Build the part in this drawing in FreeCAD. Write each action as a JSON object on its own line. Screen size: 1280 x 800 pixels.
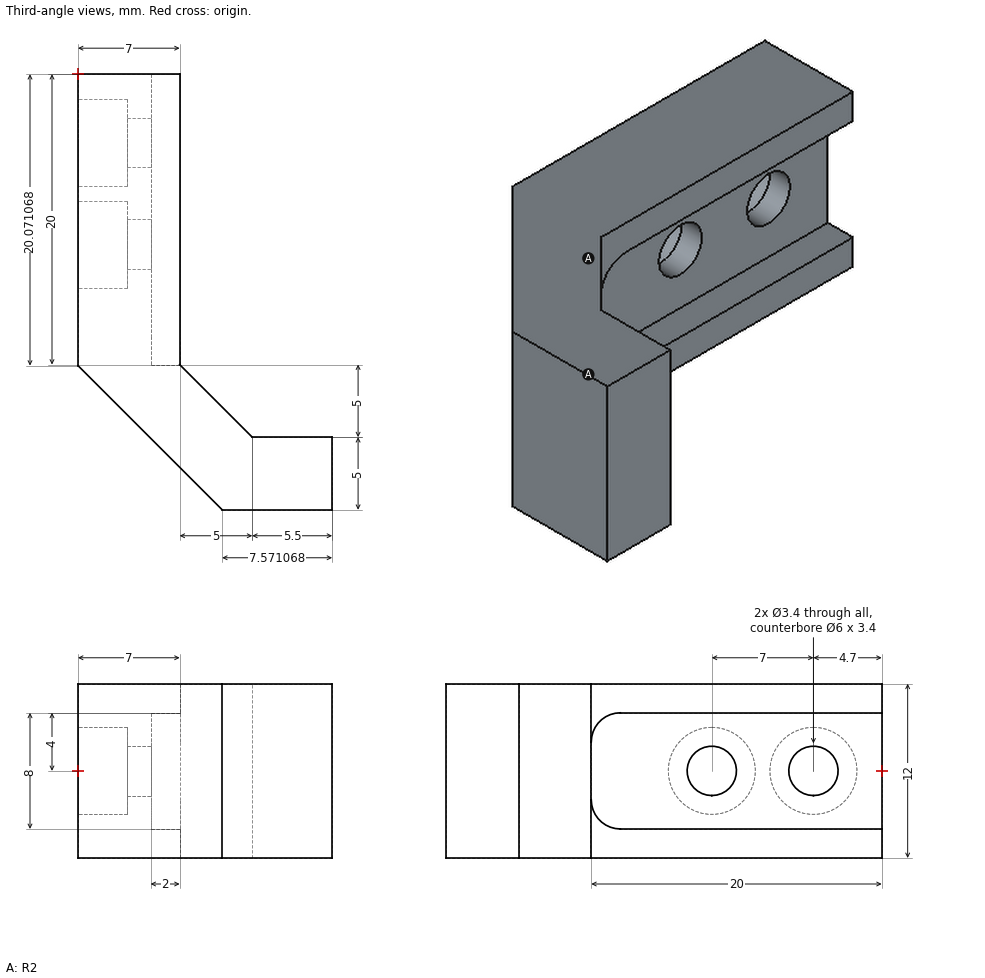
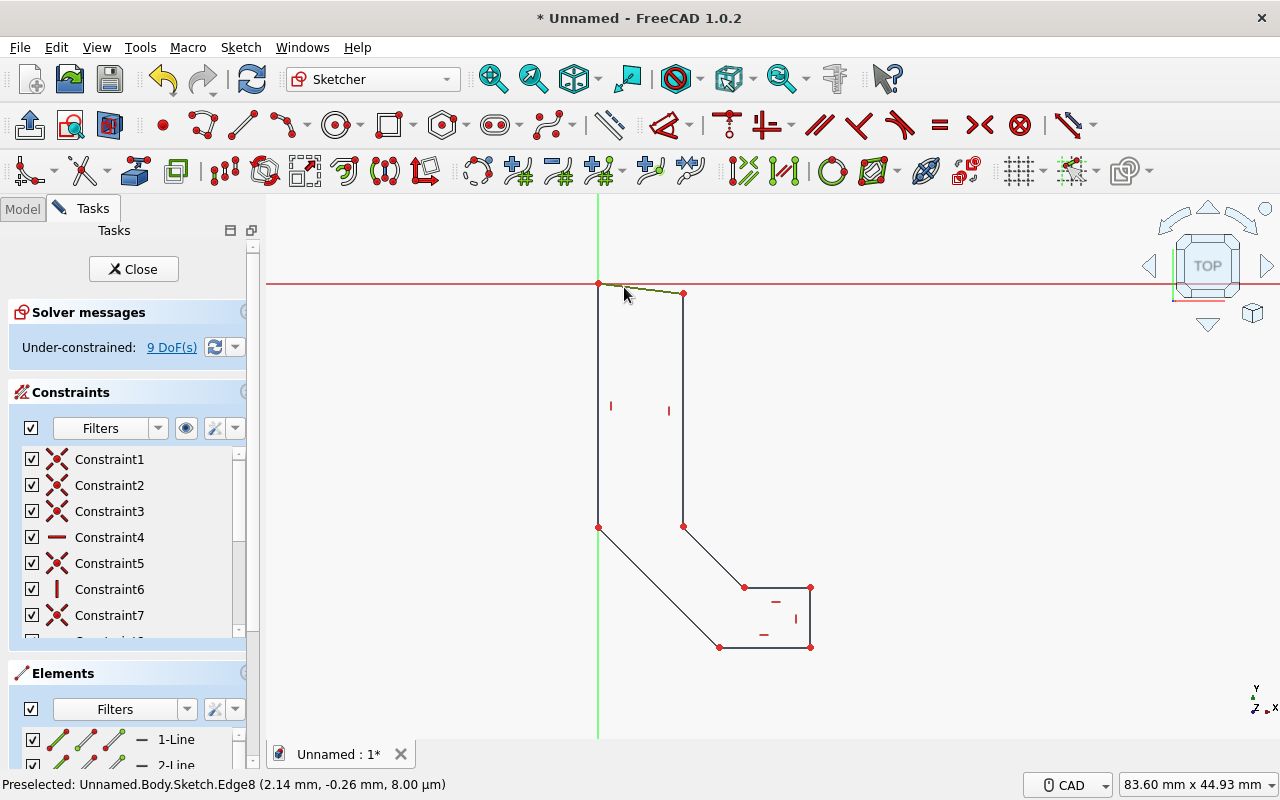
{"action": "key", "text": "h"}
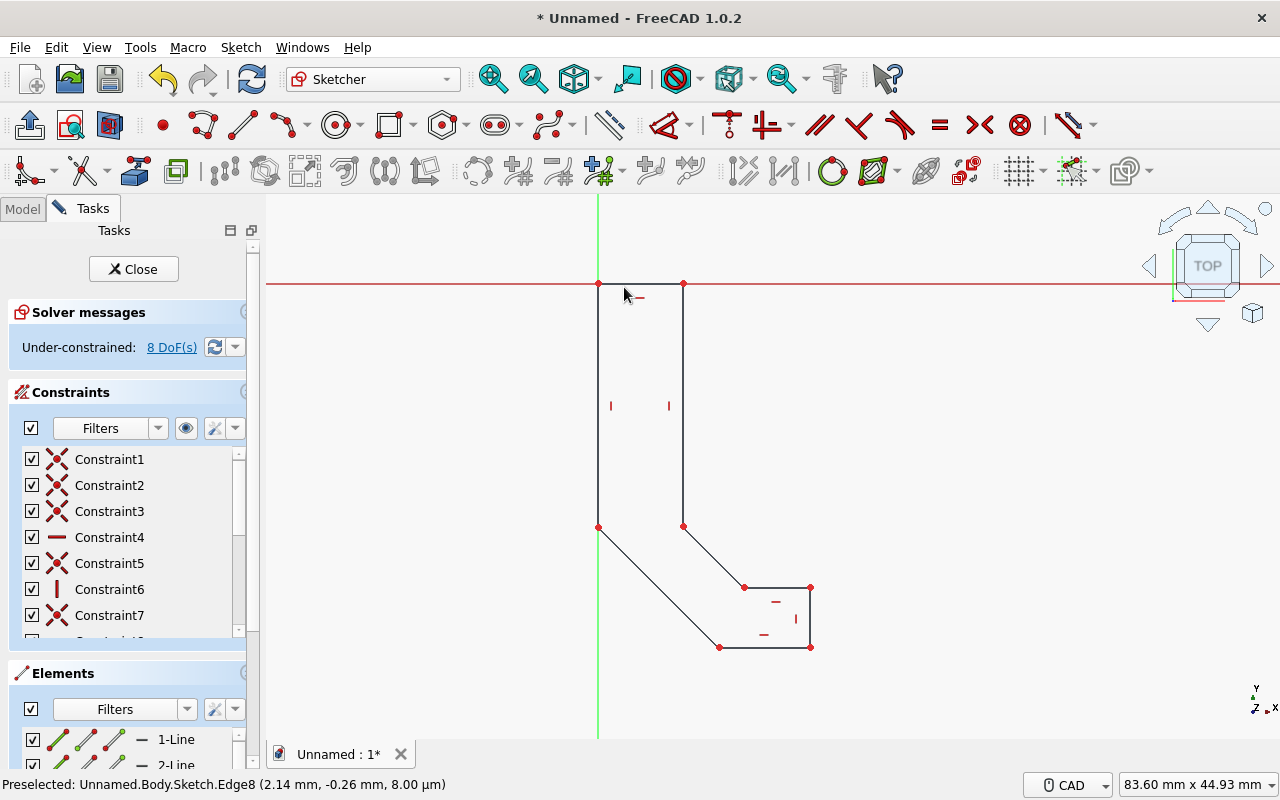
{"action": "left_click", "coordinate": [664, 126]}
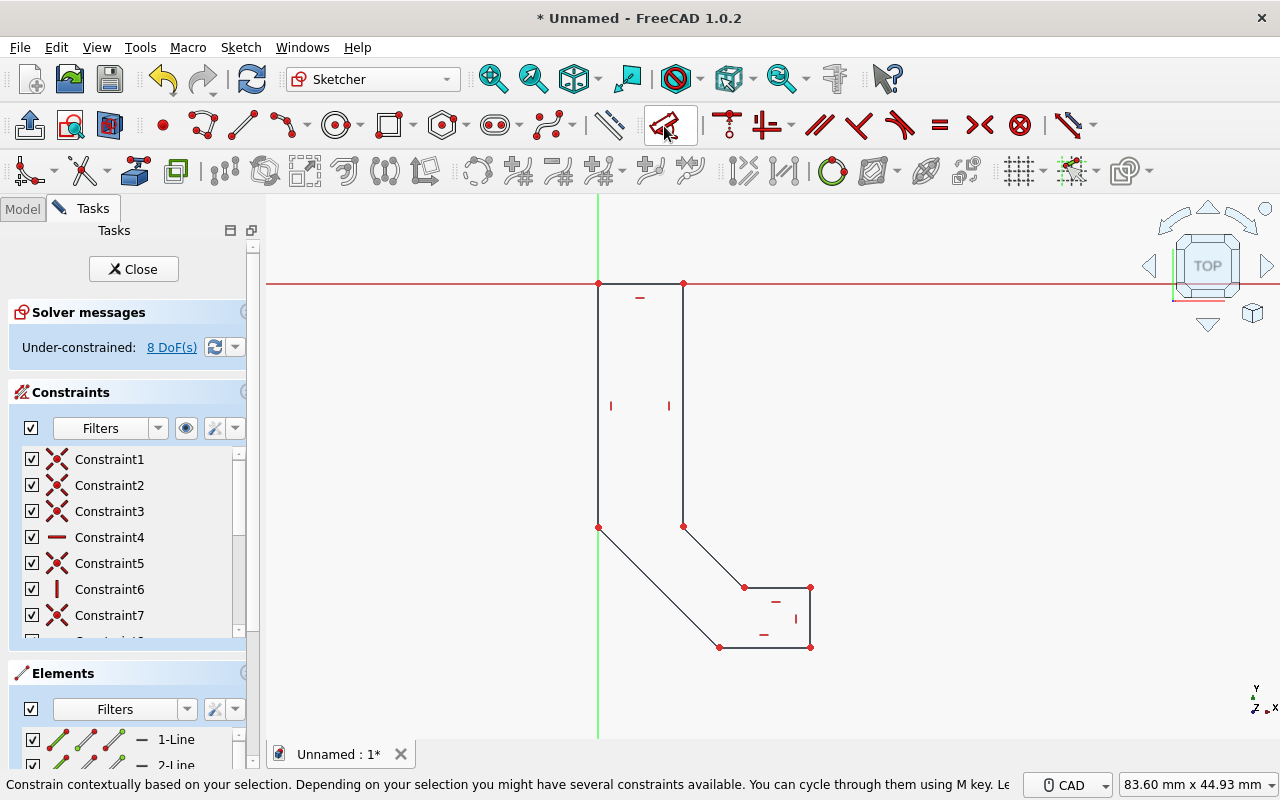
{"action": "left_click", "coordinate": [810, 630]}
{"action": "left_click", "coordinate": [844, 618]}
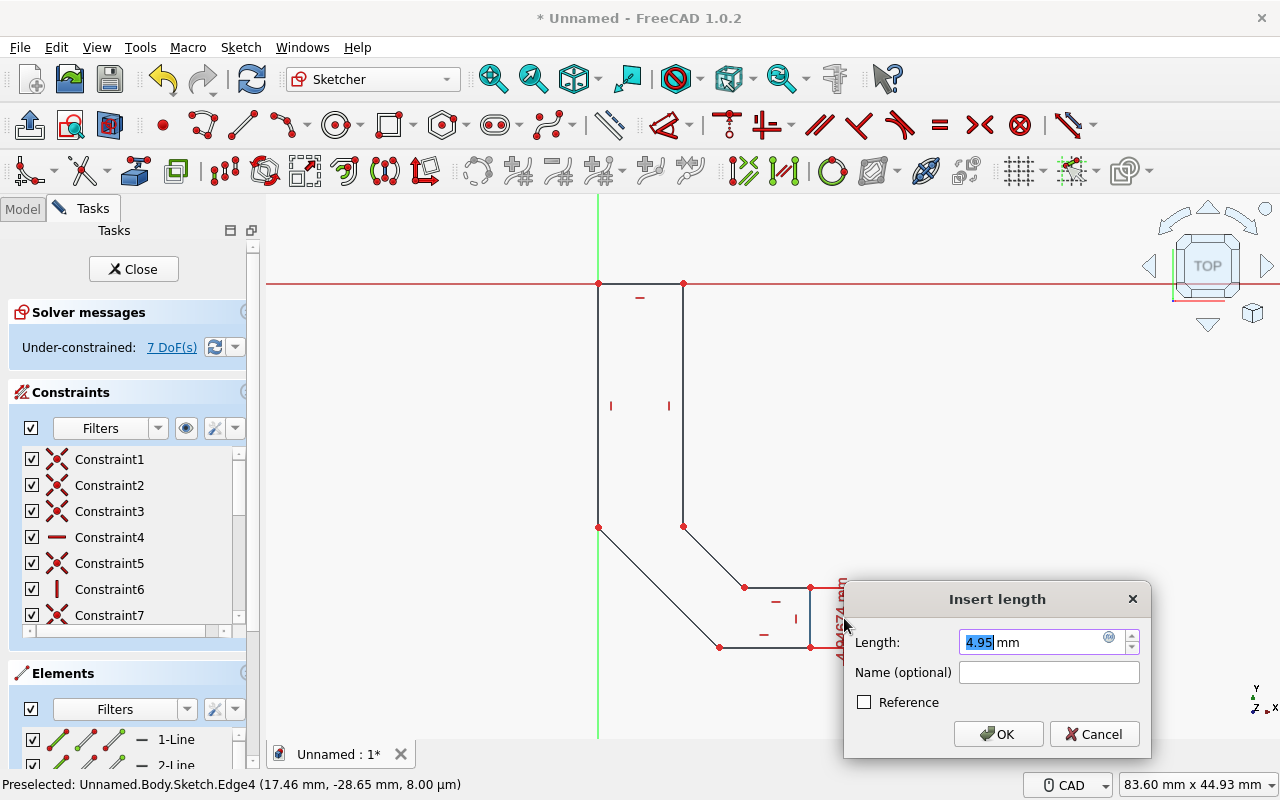
{"action": "type", "text": "5"}
{"action": "key", "text": "Return"}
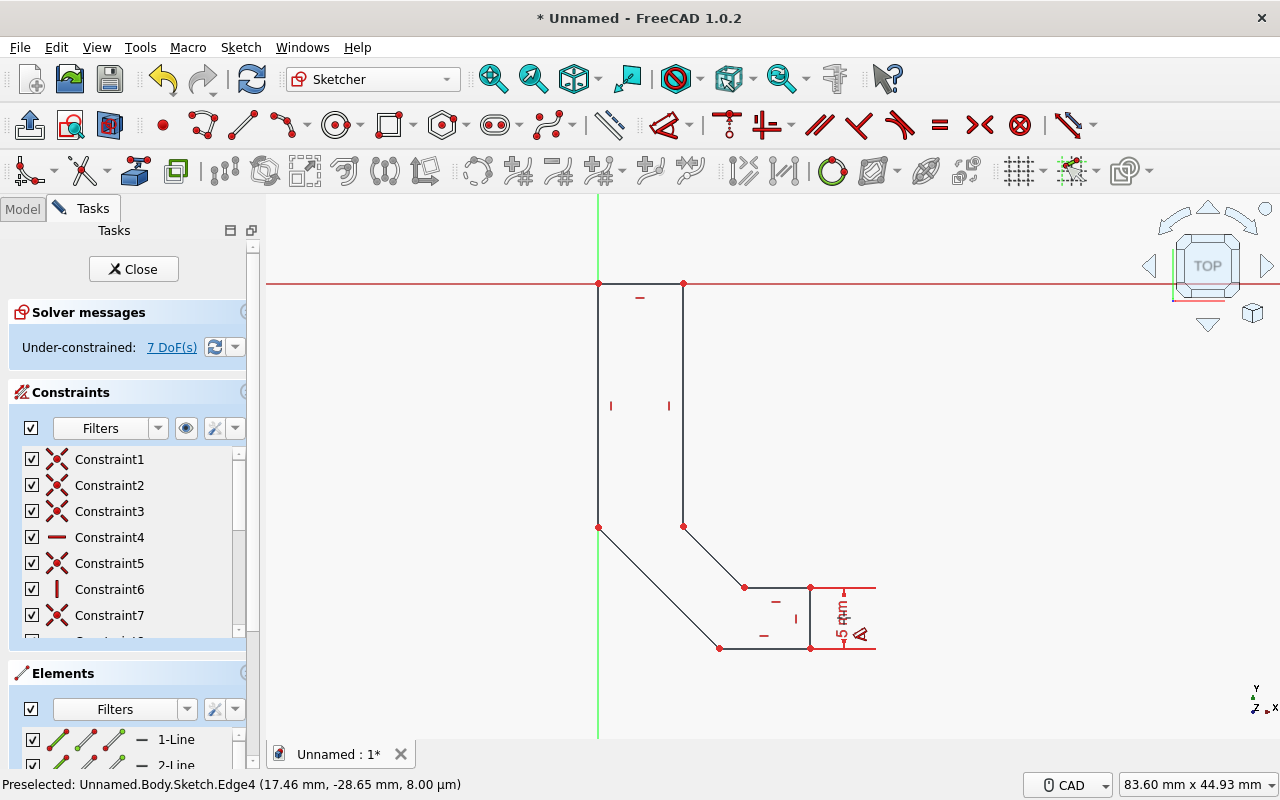
{"action": "left_click", "coordinate": [658, 284]}
{"action": "left_click", "coordinate": [641, 250]}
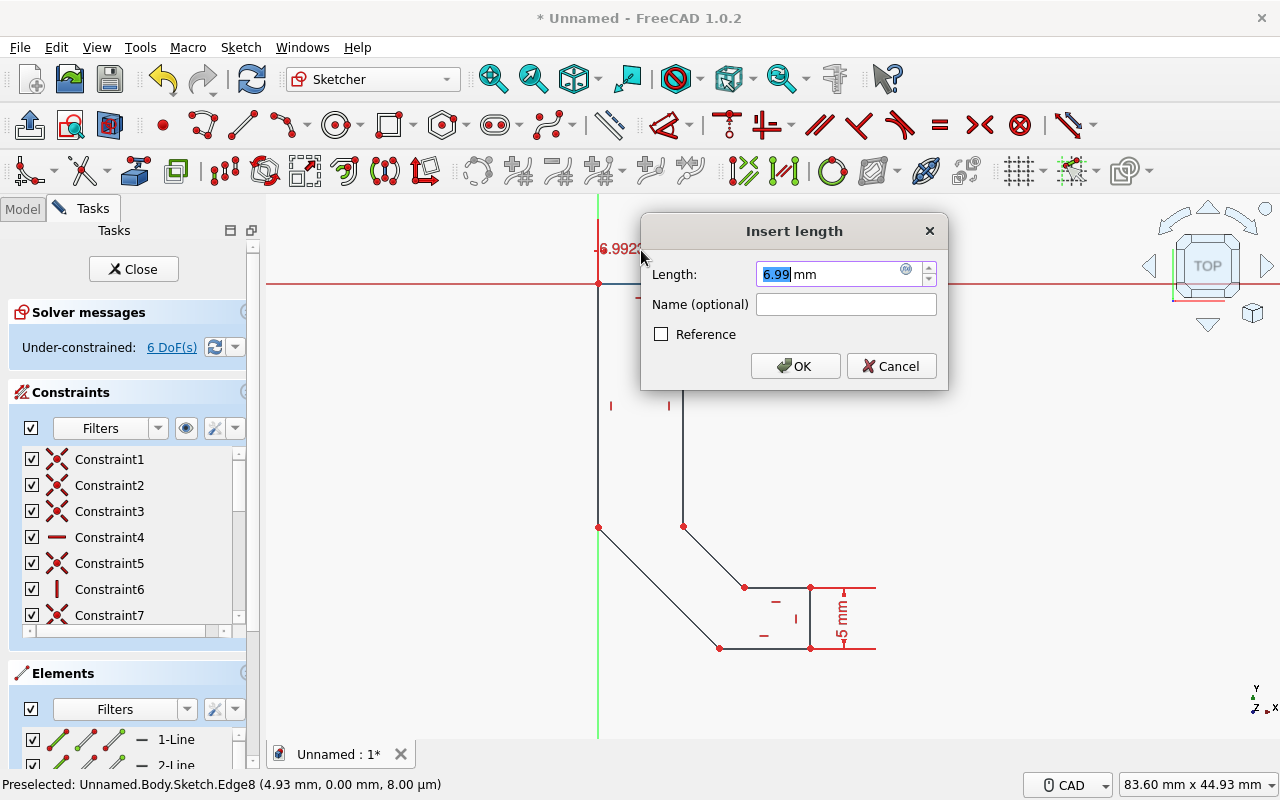
{"action": "type", "text": "7"}
{"action": "key", "text": "Return"}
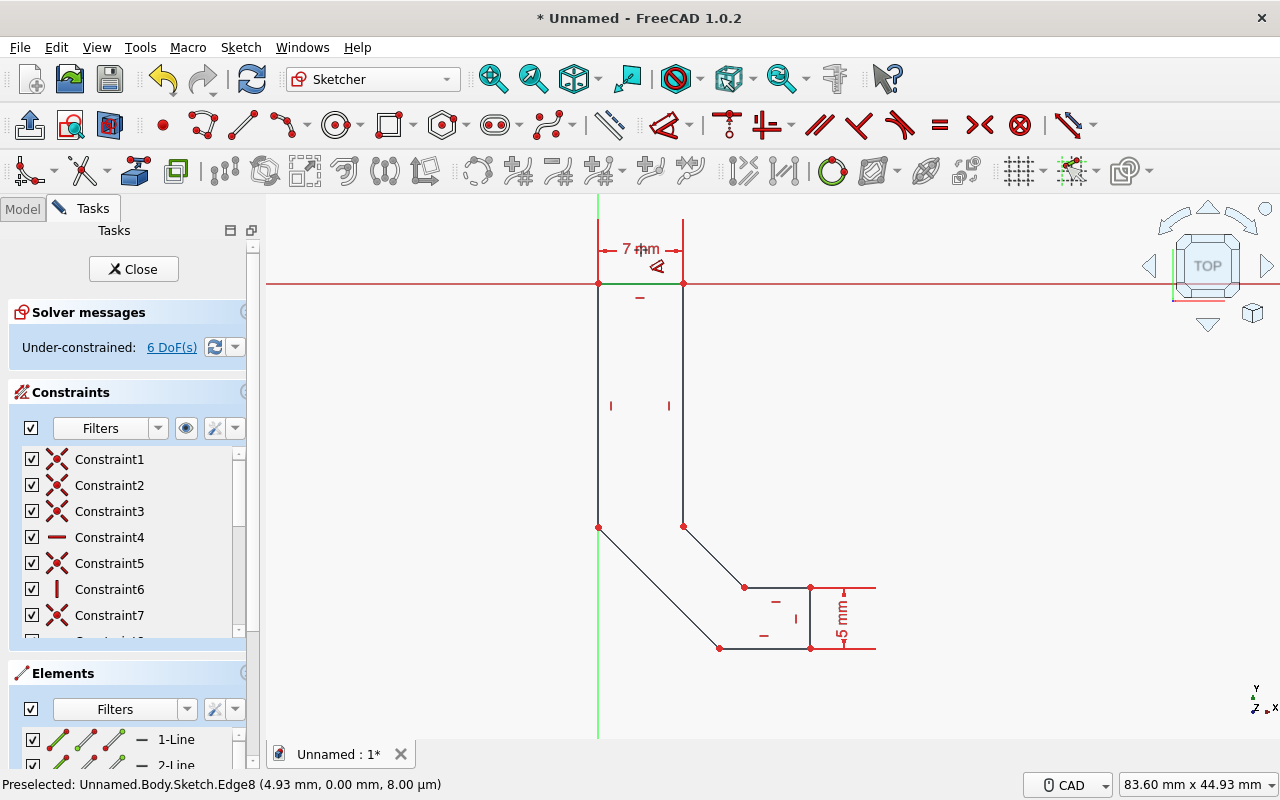
{"action": "left_click", "coordinate": [683, 454]}
{"action": "left_click", "coordinate": [649, 405]}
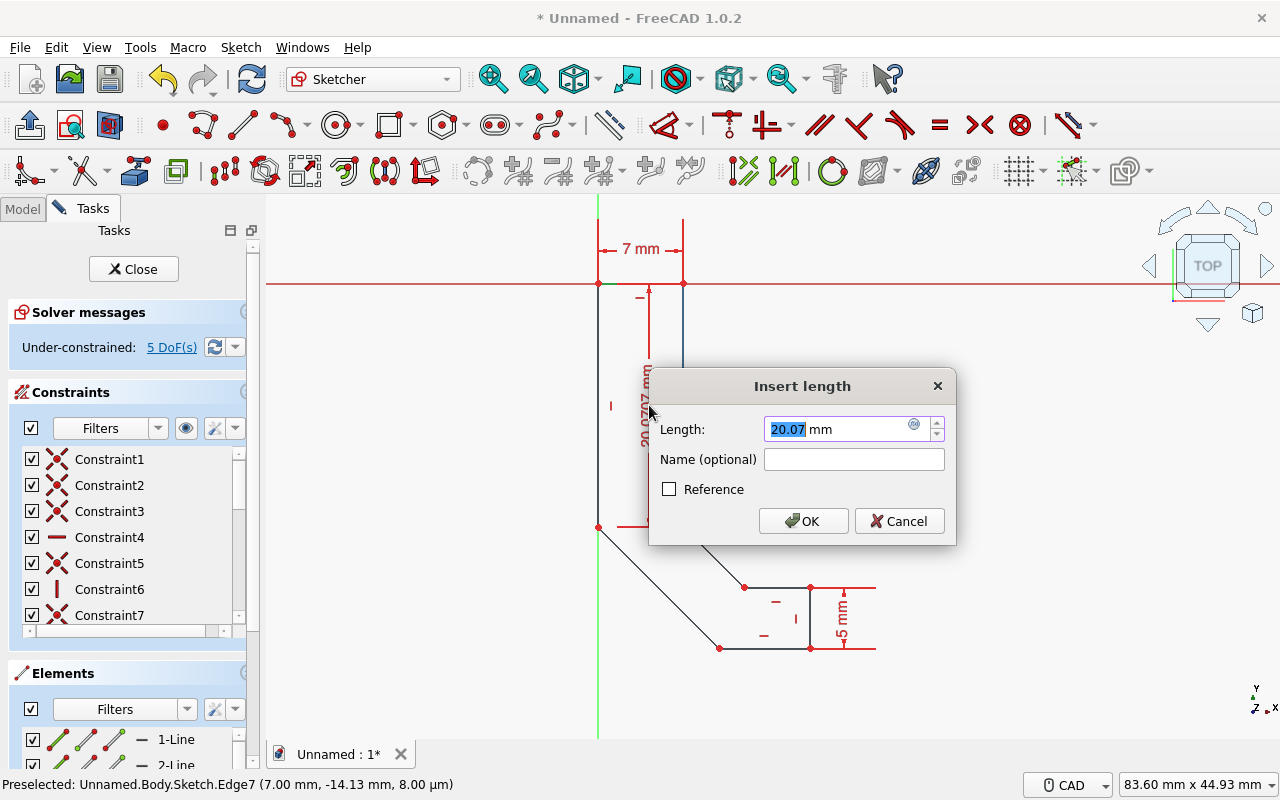
{"action": "type", "text": "20"}
{"action": "key", "text": "Return"}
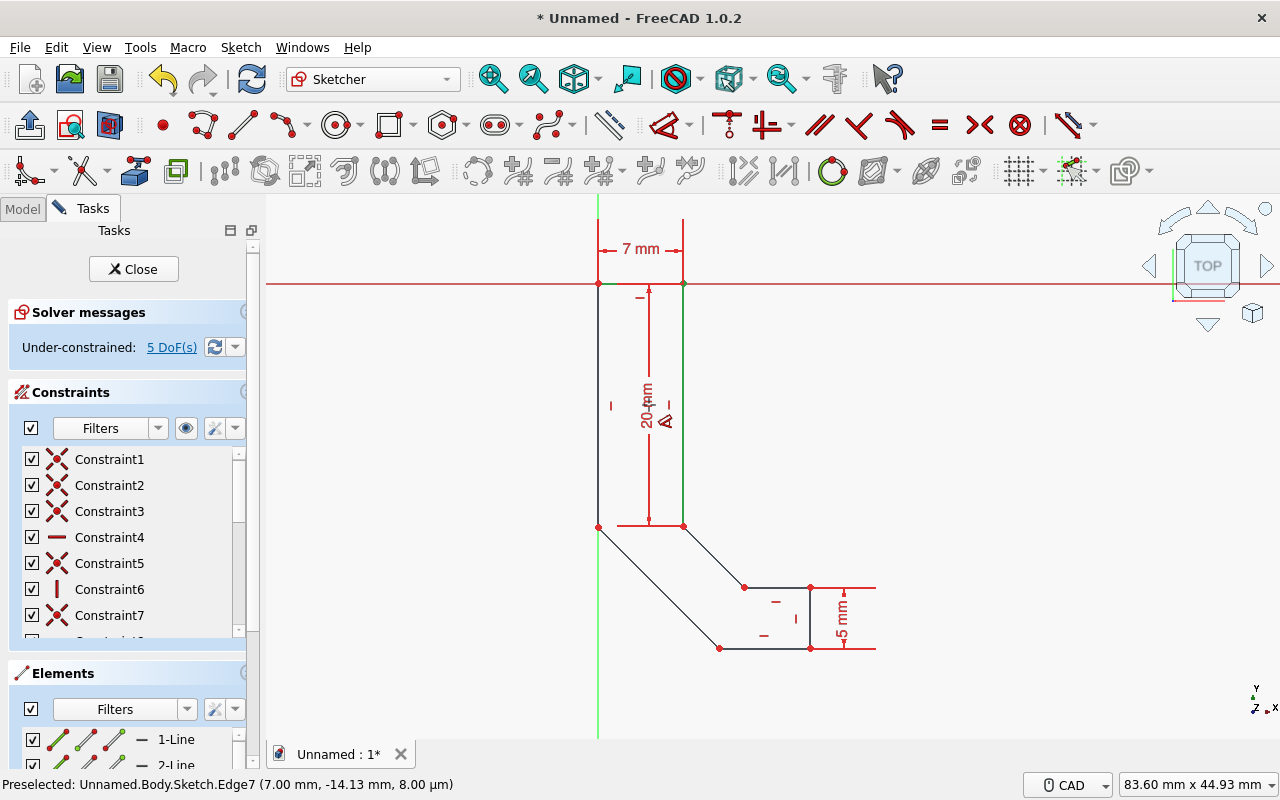
{"action": "left_click", "coordinate": [726, 569]}
{"action": "left_click", "coordinate": [714, 622]}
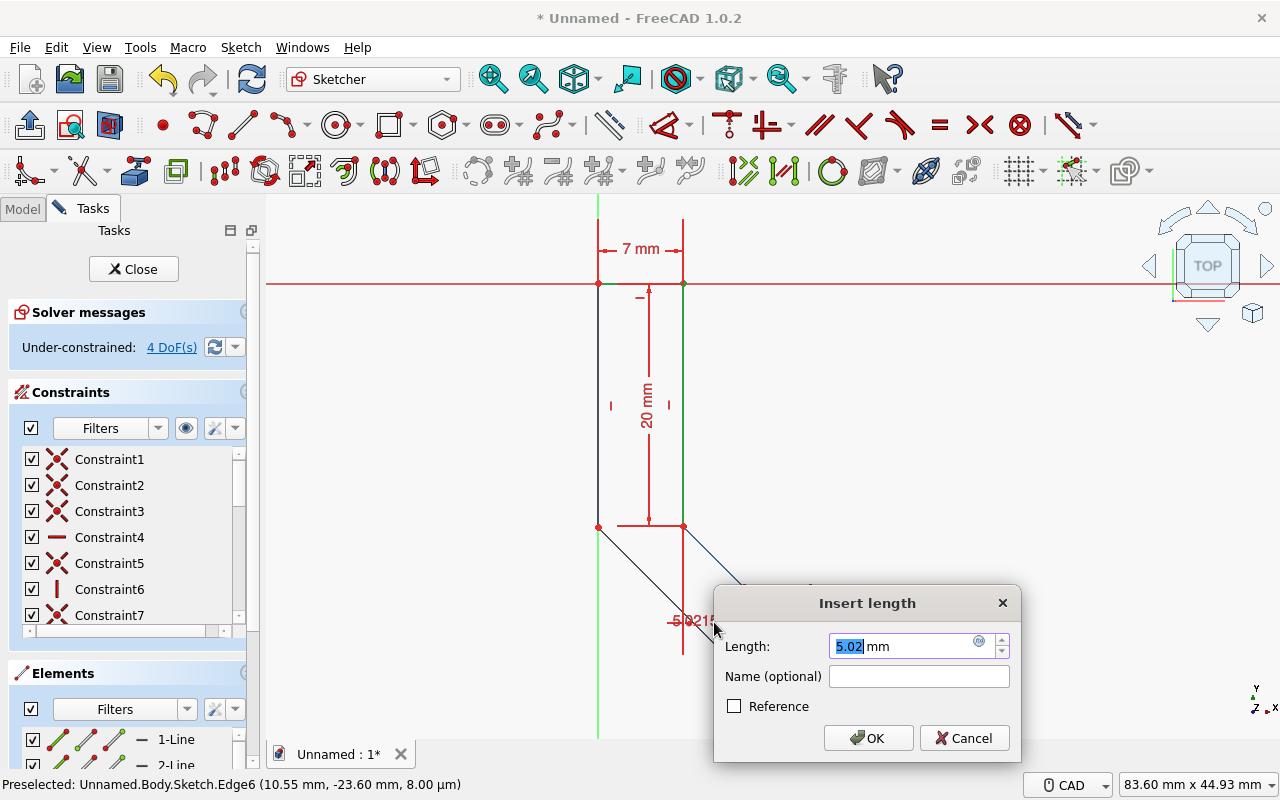
{"action": "type", "text": "5"}
{"action": "key", "text": "Return"}